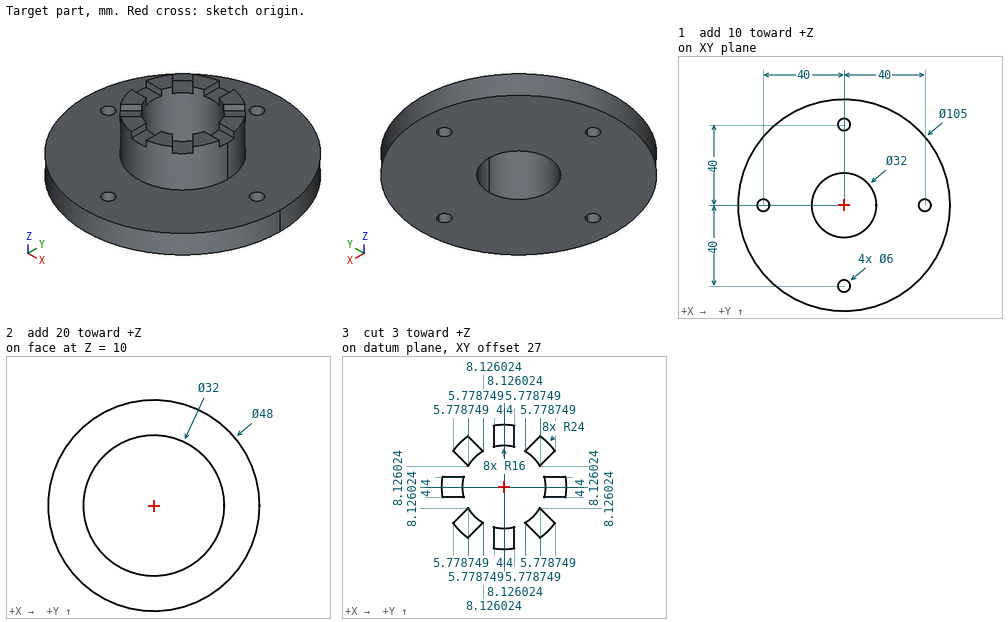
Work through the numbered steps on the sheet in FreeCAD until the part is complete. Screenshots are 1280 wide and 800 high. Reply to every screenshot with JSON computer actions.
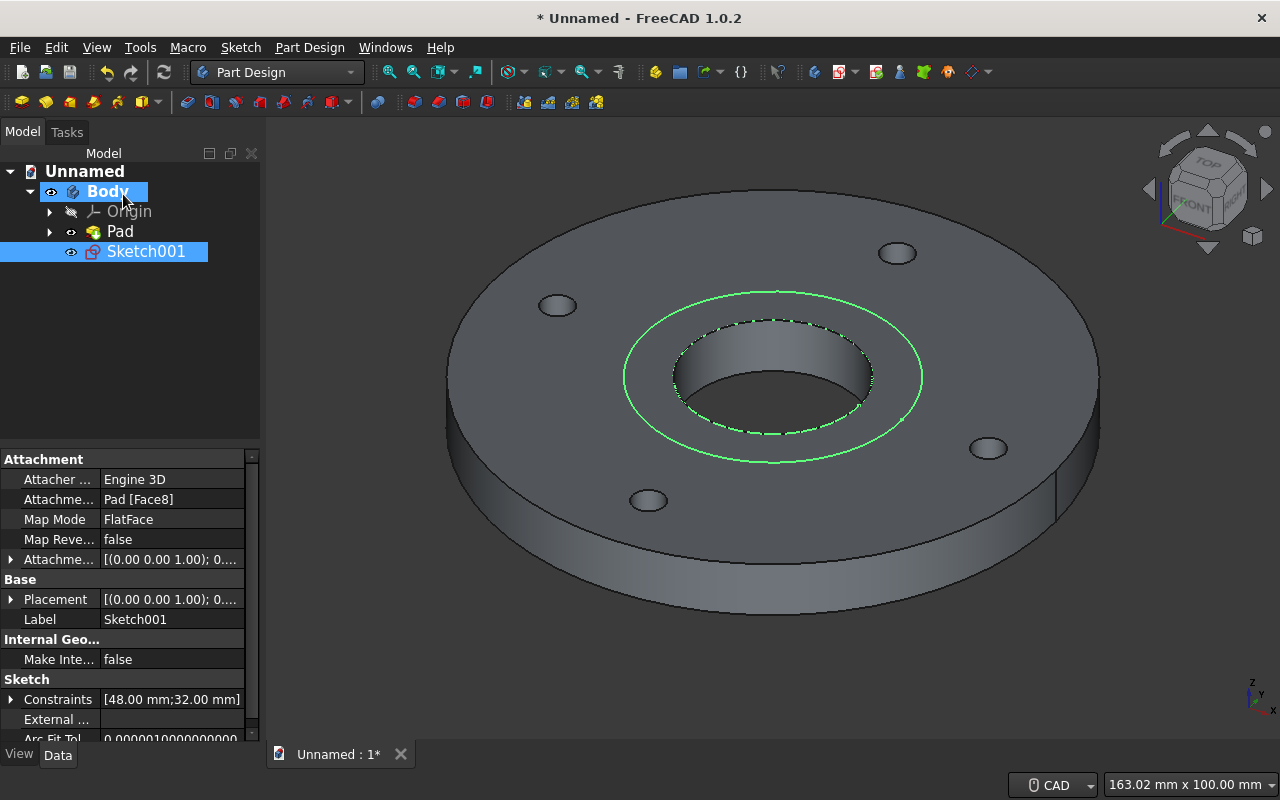
{"action": "left_click", "coordinate": [22, 102]}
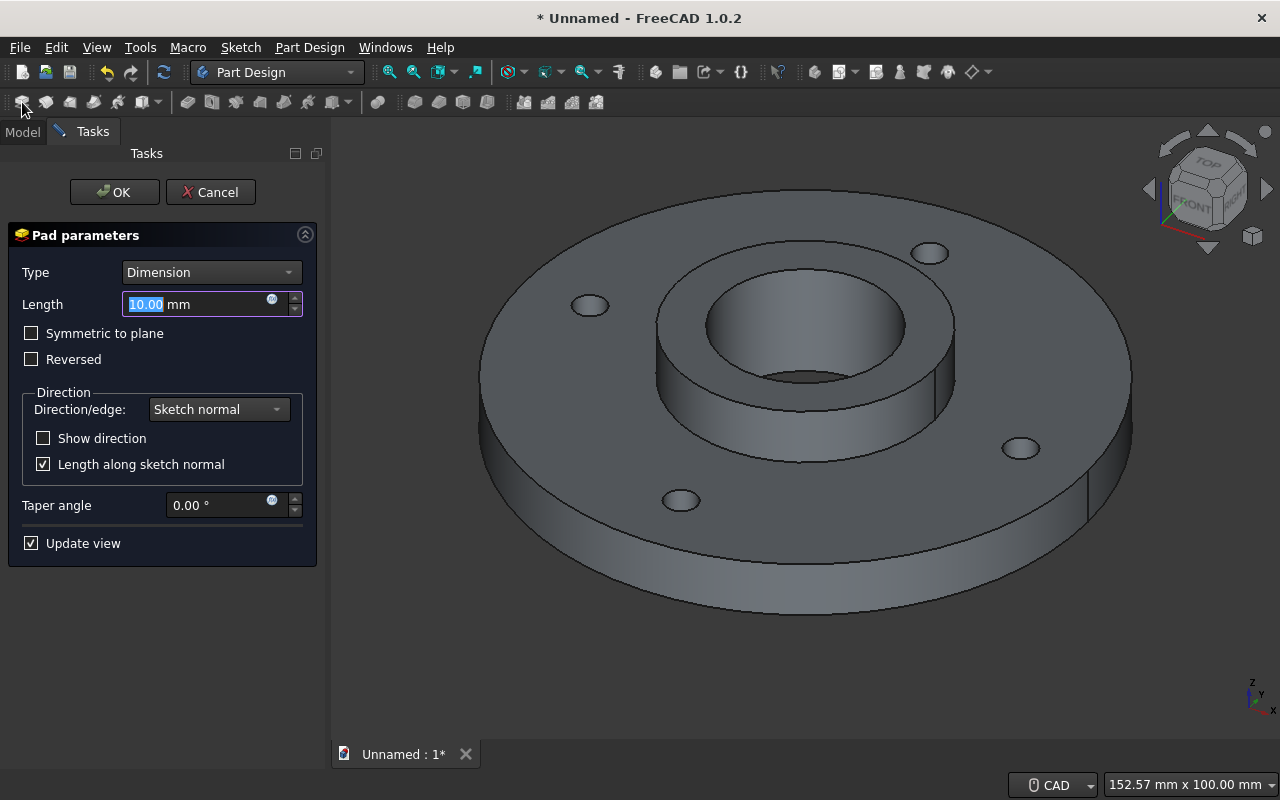
{"action": "type", "text": "20"}
{"action": "key", "text": "Tab"}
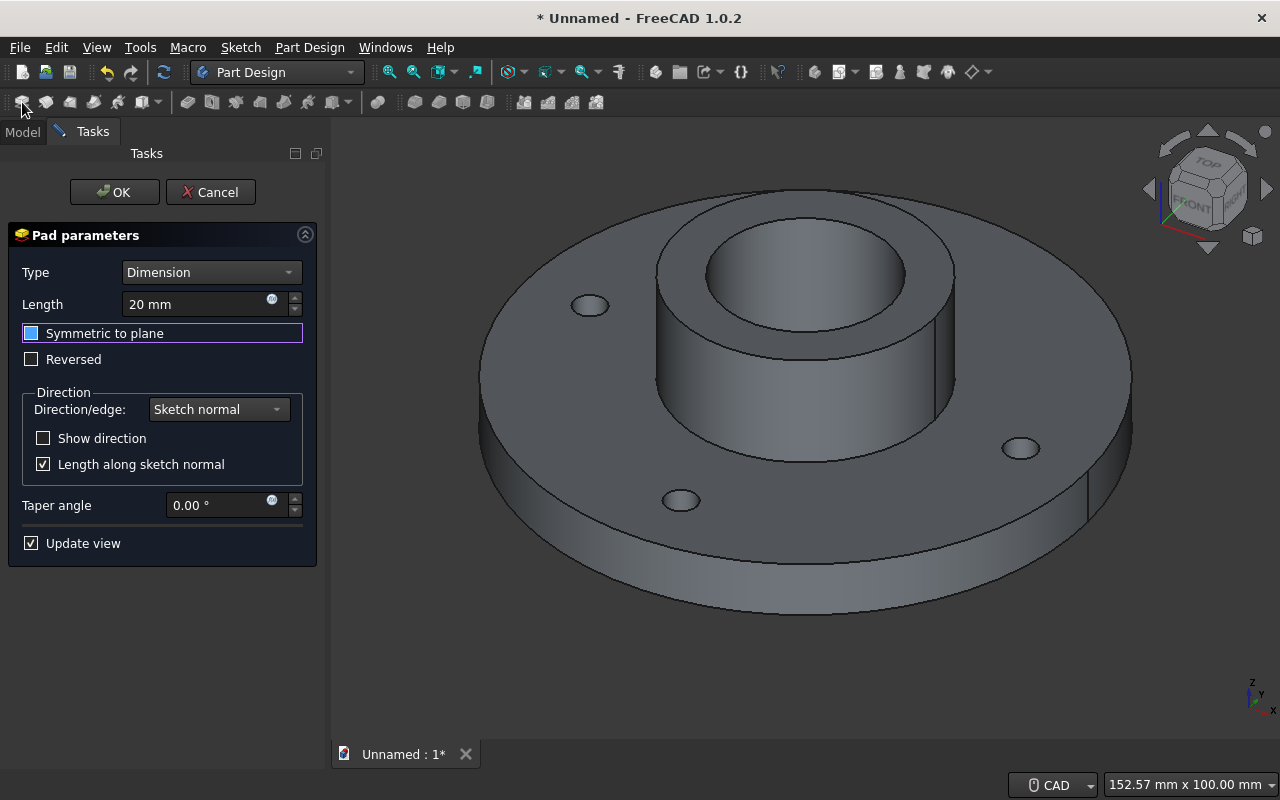
{"action": "left_click", "coordinate": [115, 192]}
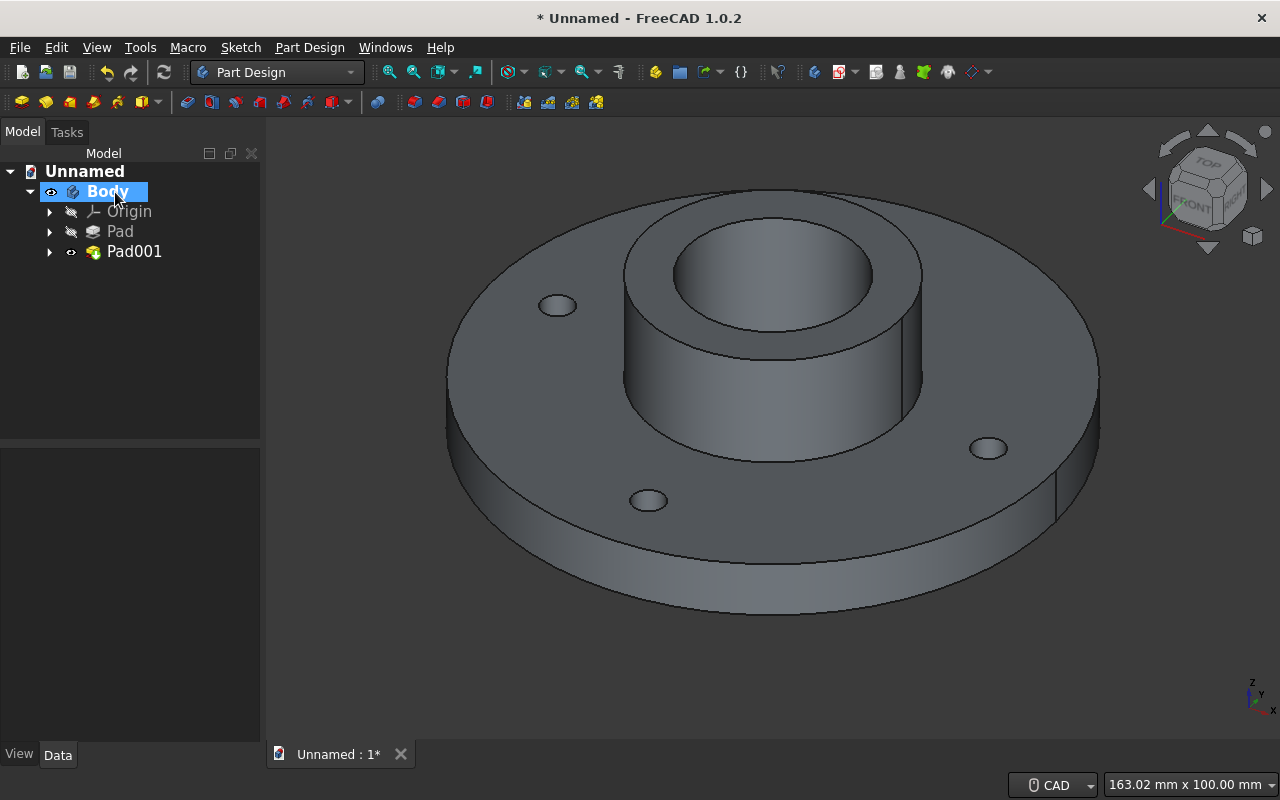
{"action": "left_click", "coordinate": [390, 72]}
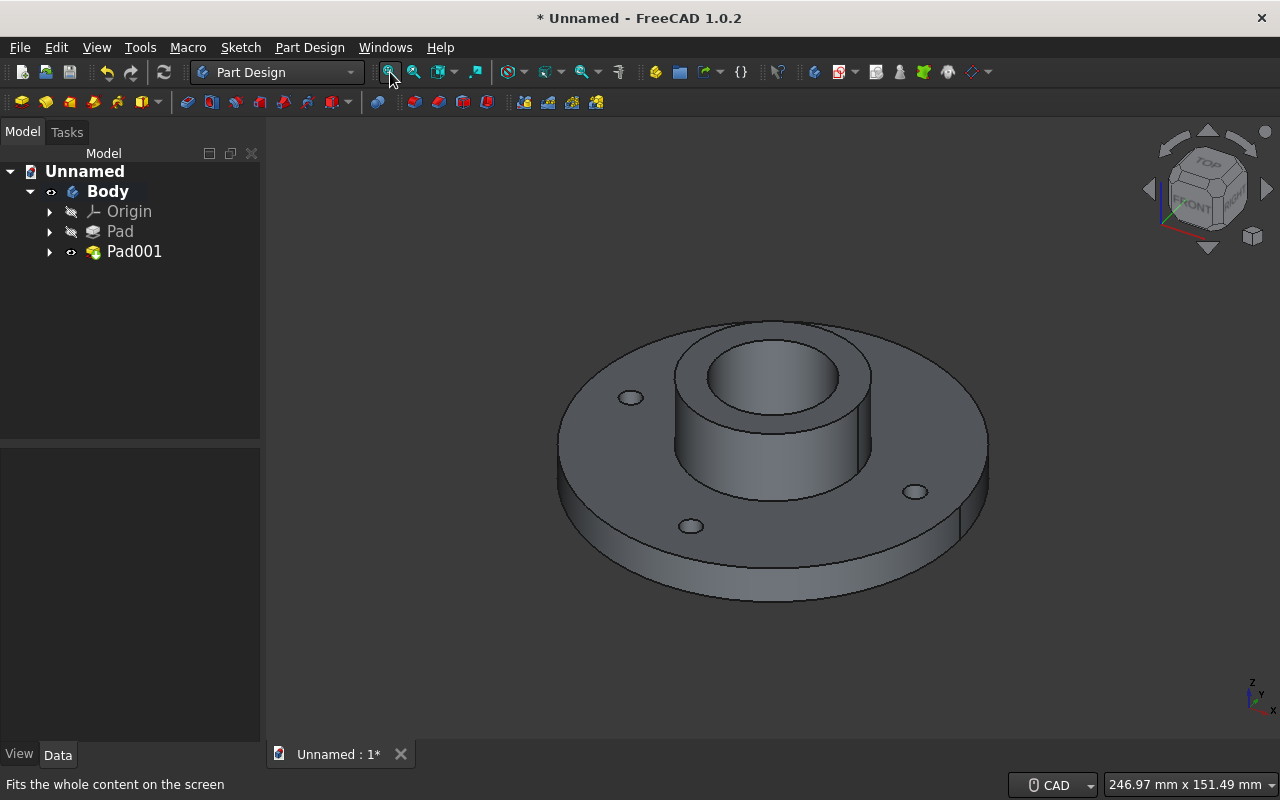
{"action": "left_click", "coordinate": [50, 212]}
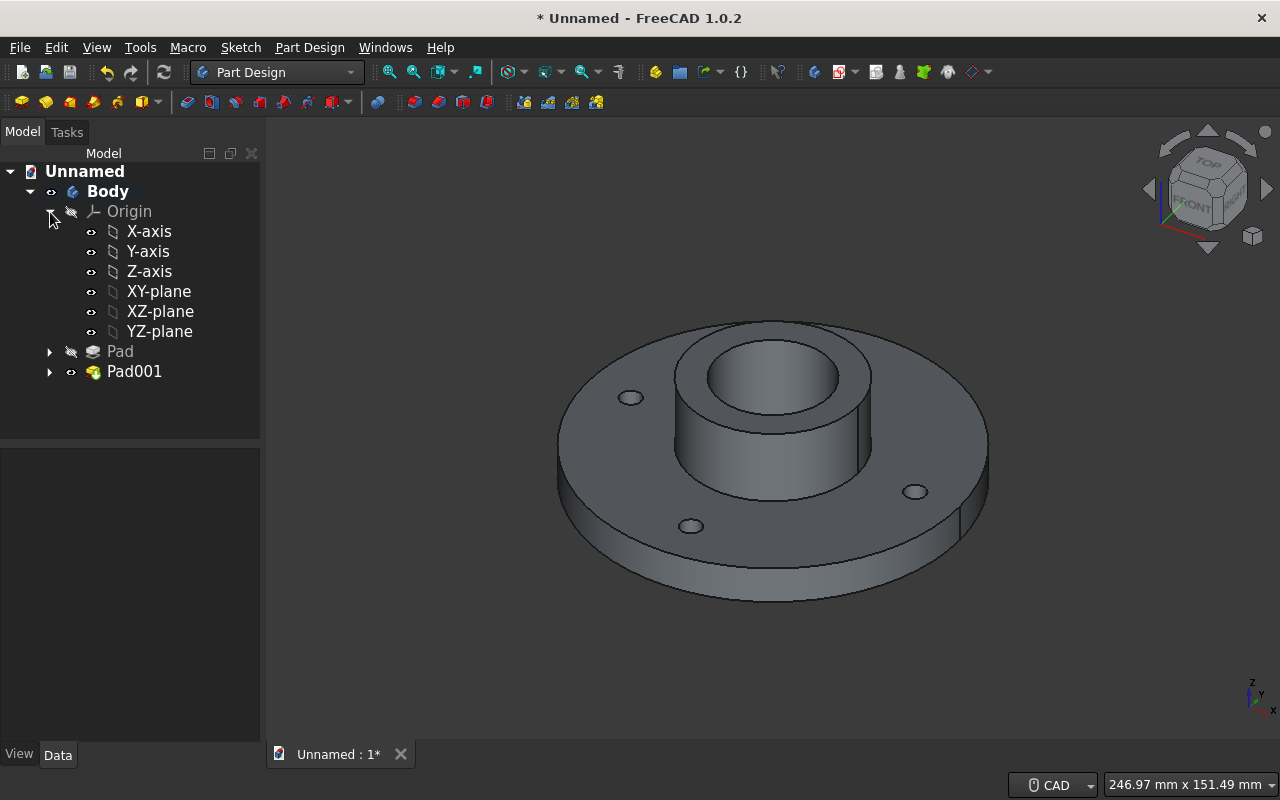
{"action": "left_click", "coordinate": [136, 292]}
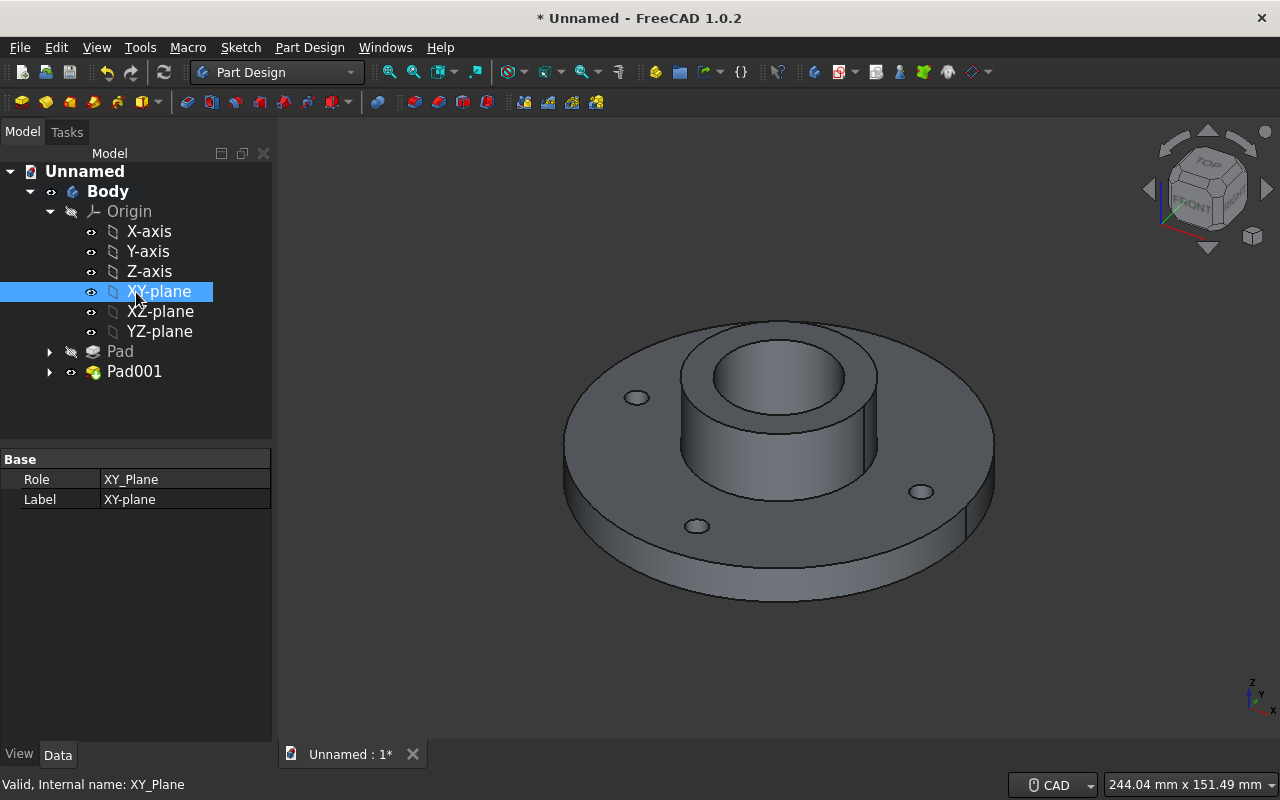
{"action": "left_click", "coordinate": [972, 72]}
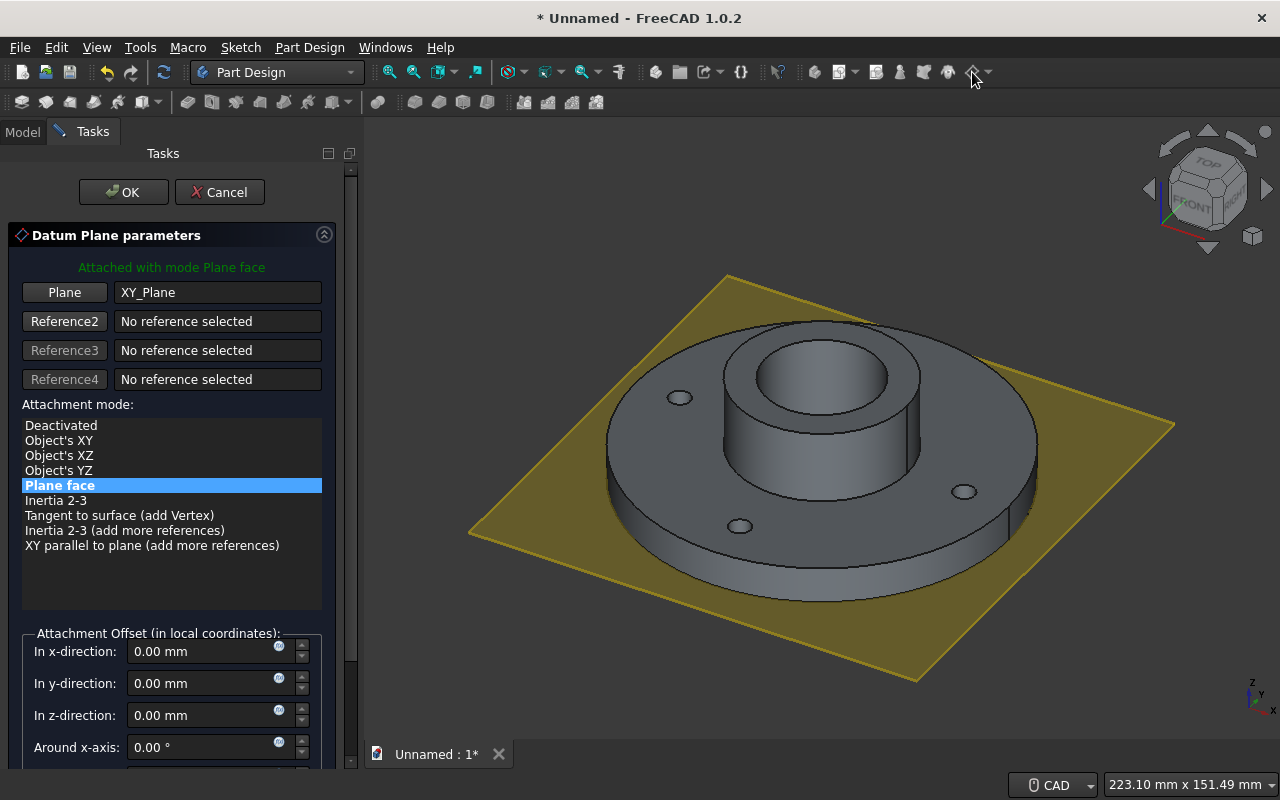
{"action": "triple_click", "coordinate": [210, 715]}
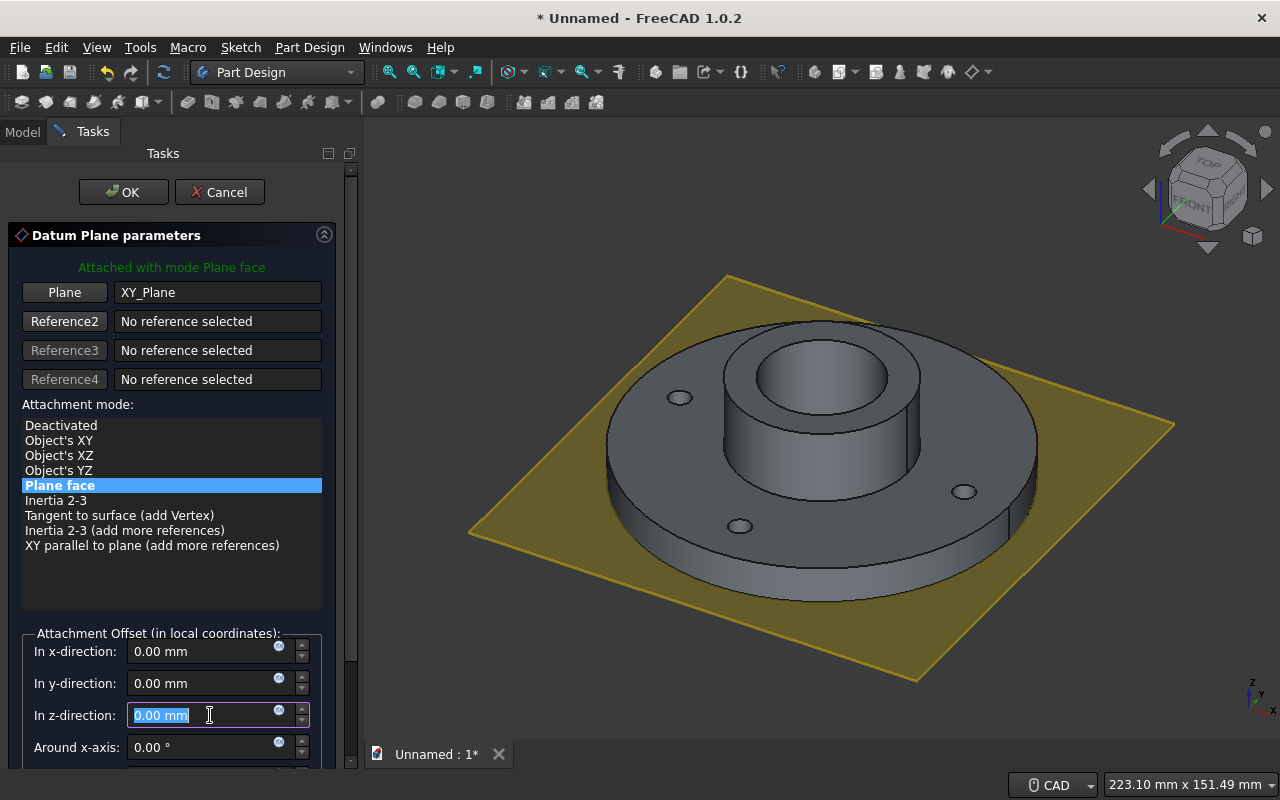
{"action": "type", "text": "27"}
{"action": "key", "text": "Tab"}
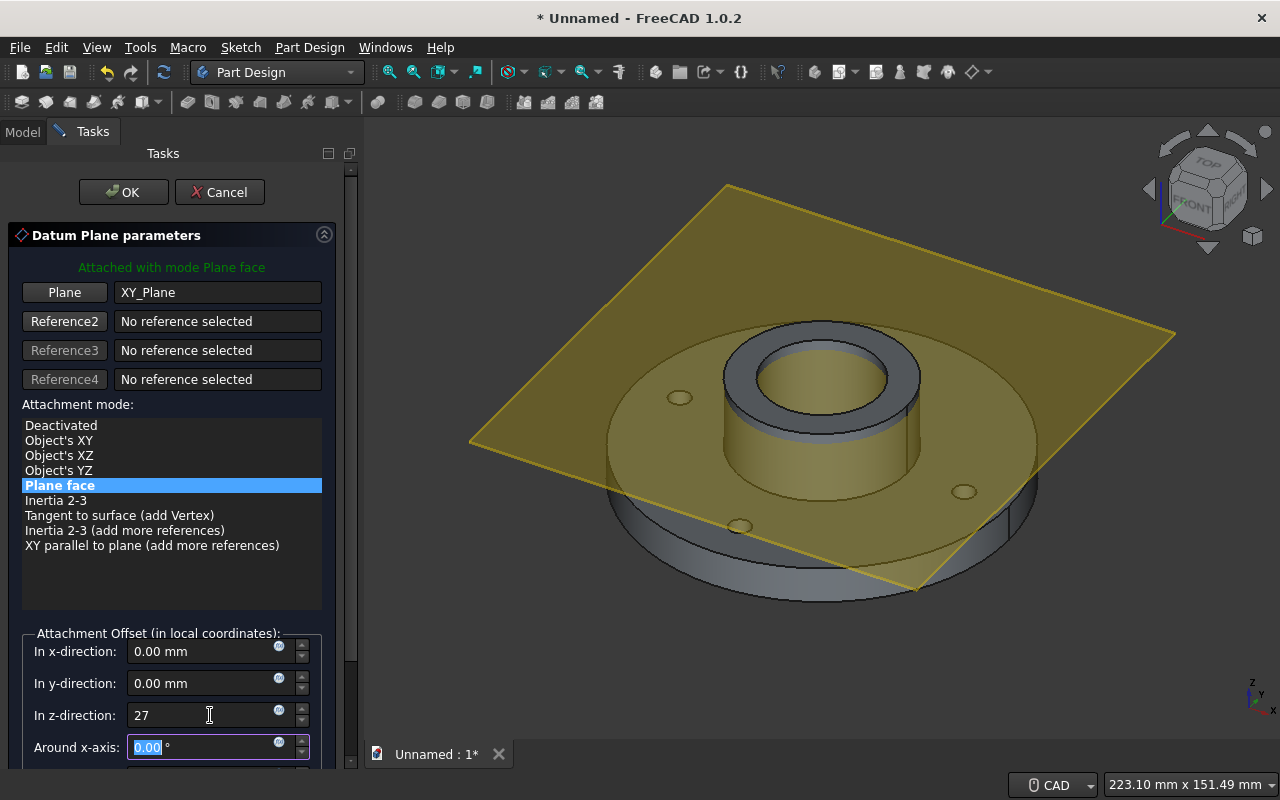
{"action": "left_click", "coordinate": [124, 192]}